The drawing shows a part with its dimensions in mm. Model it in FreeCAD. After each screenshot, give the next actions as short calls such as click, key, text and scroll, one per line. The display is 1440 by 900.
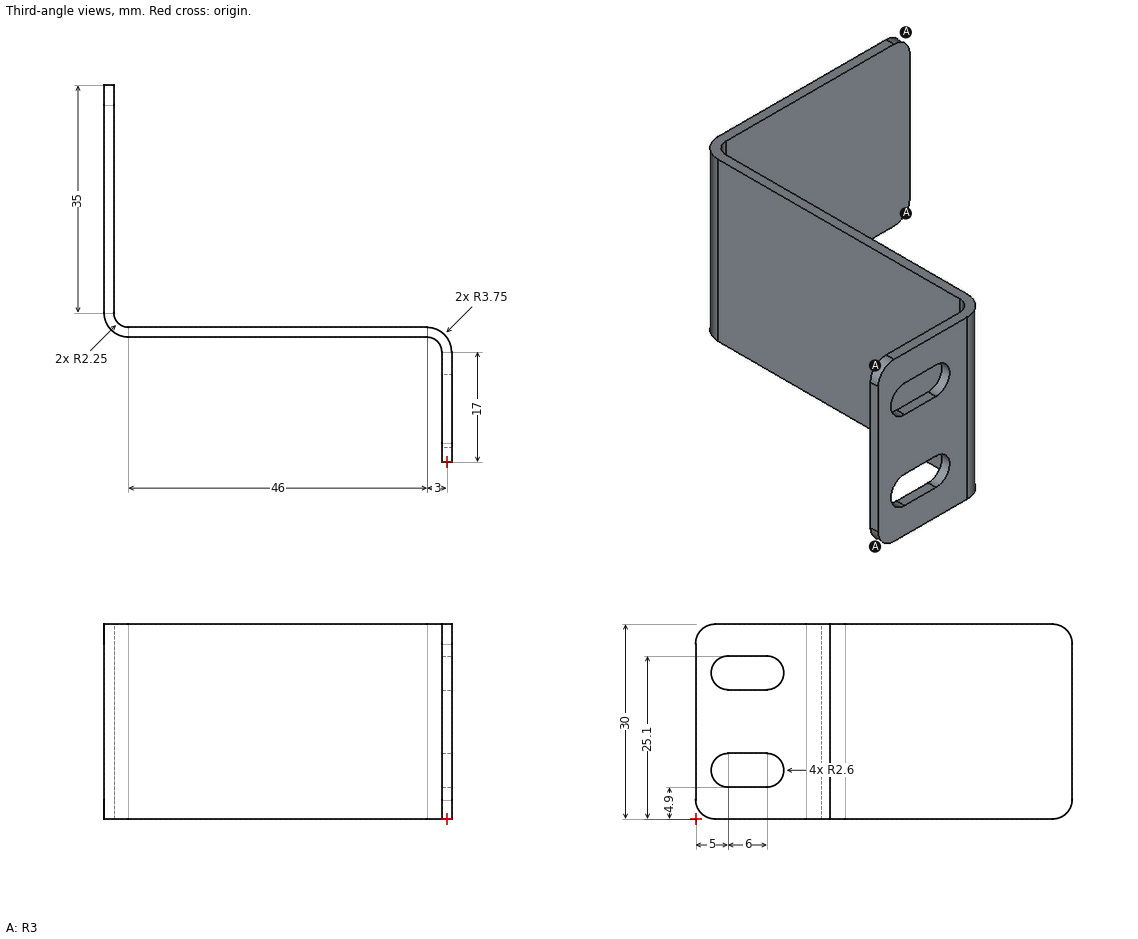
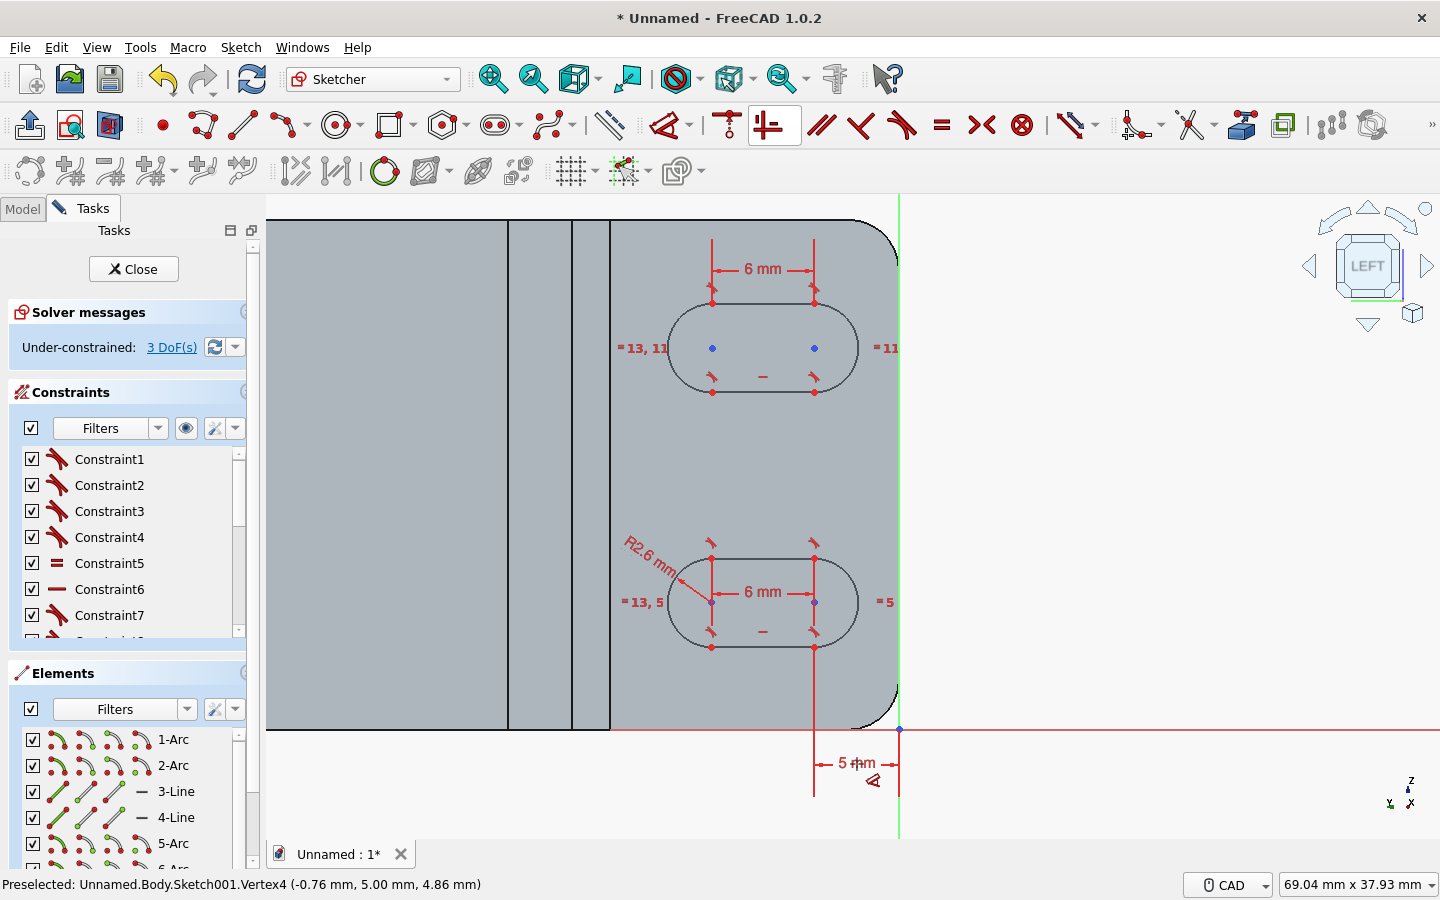
click(814, 392)
click(837, 358)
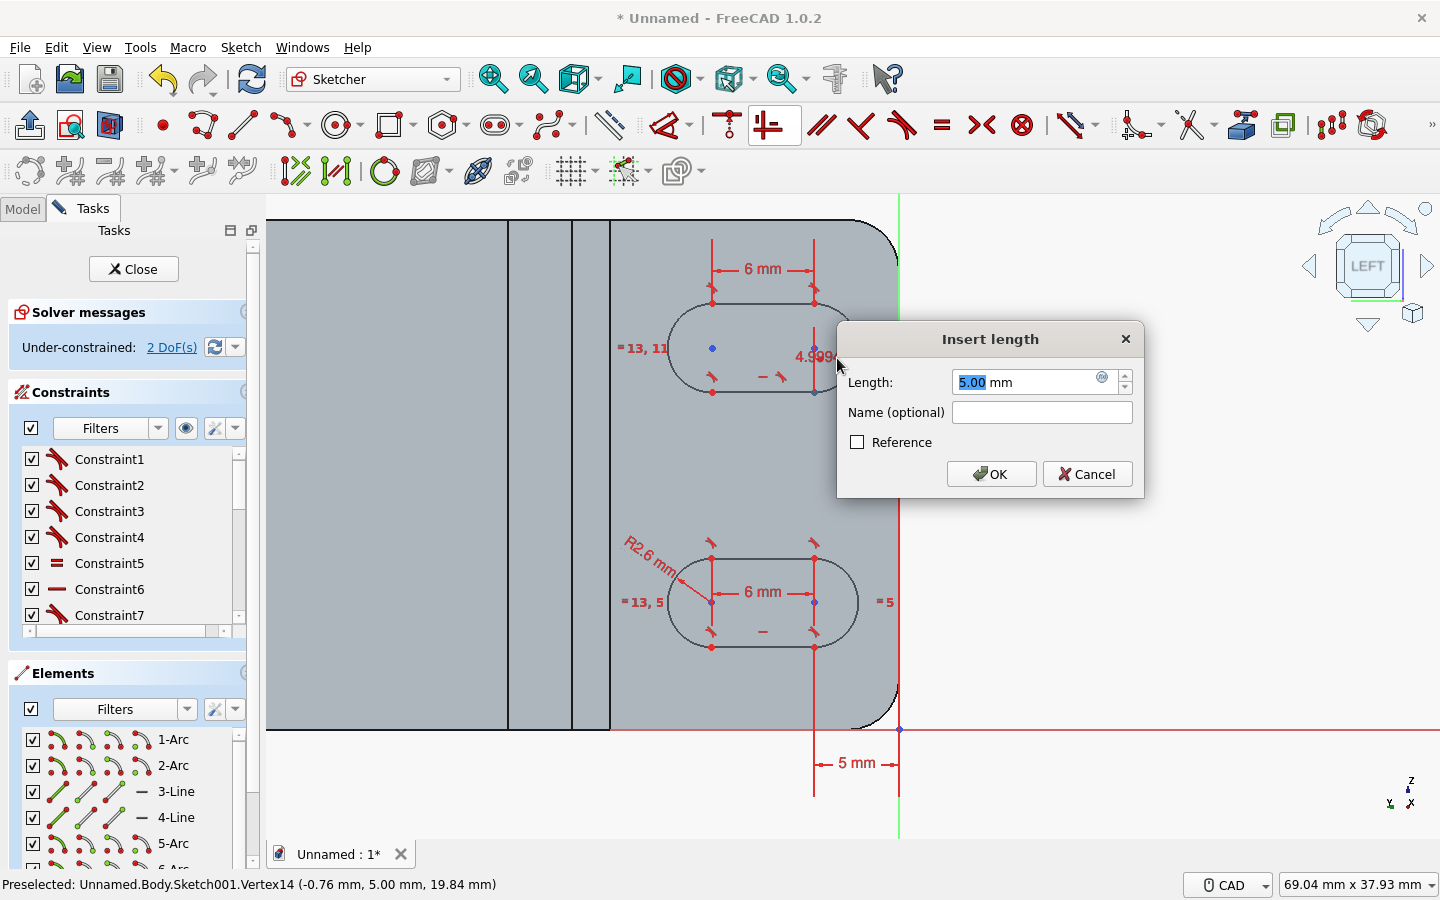
text(5)
key(Return)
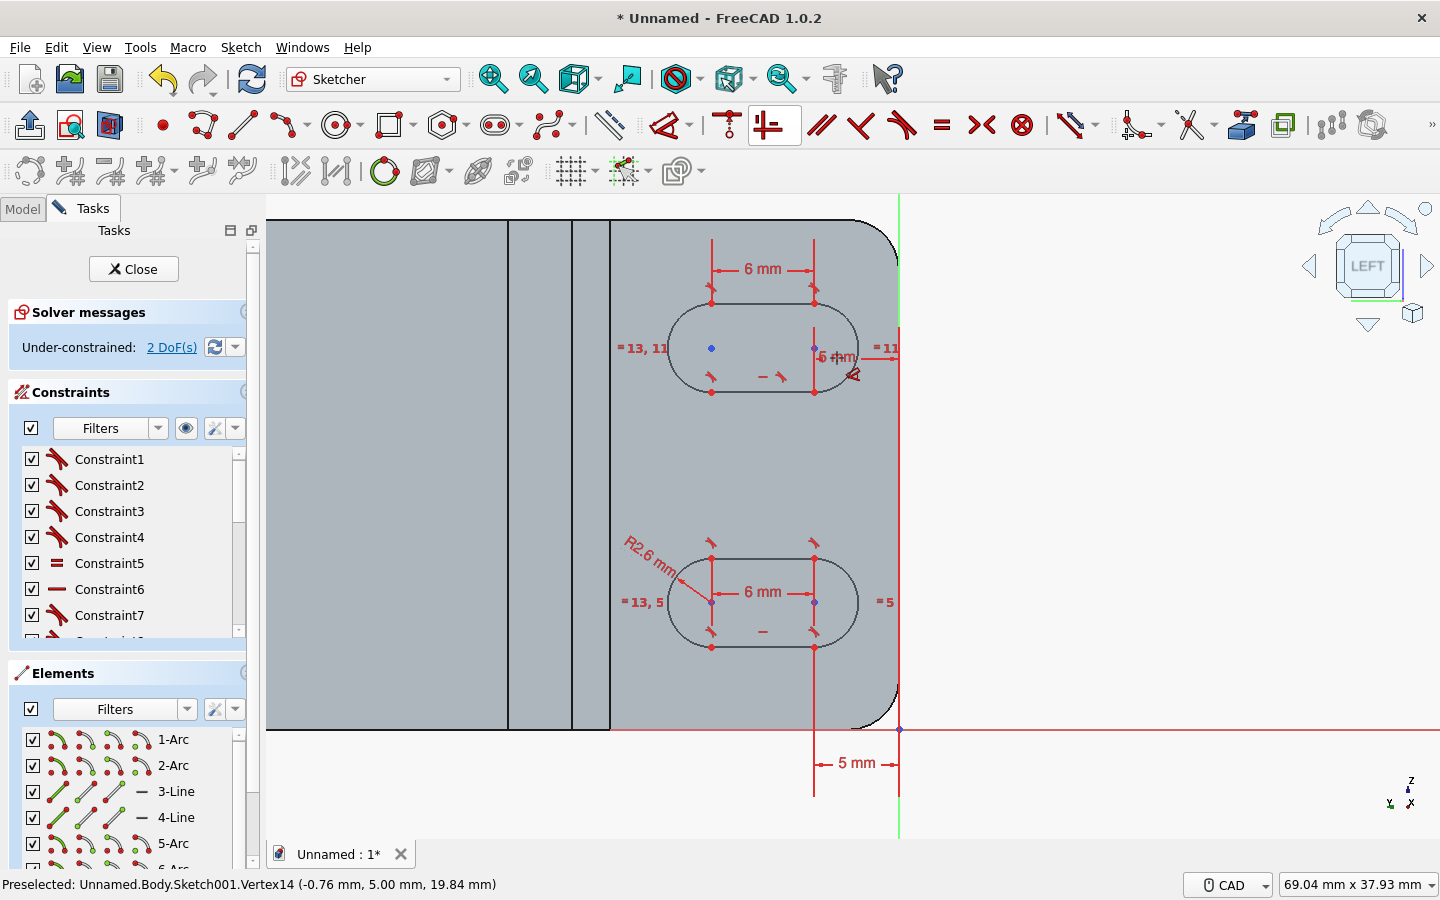
click(712, 647)
click(933, 689)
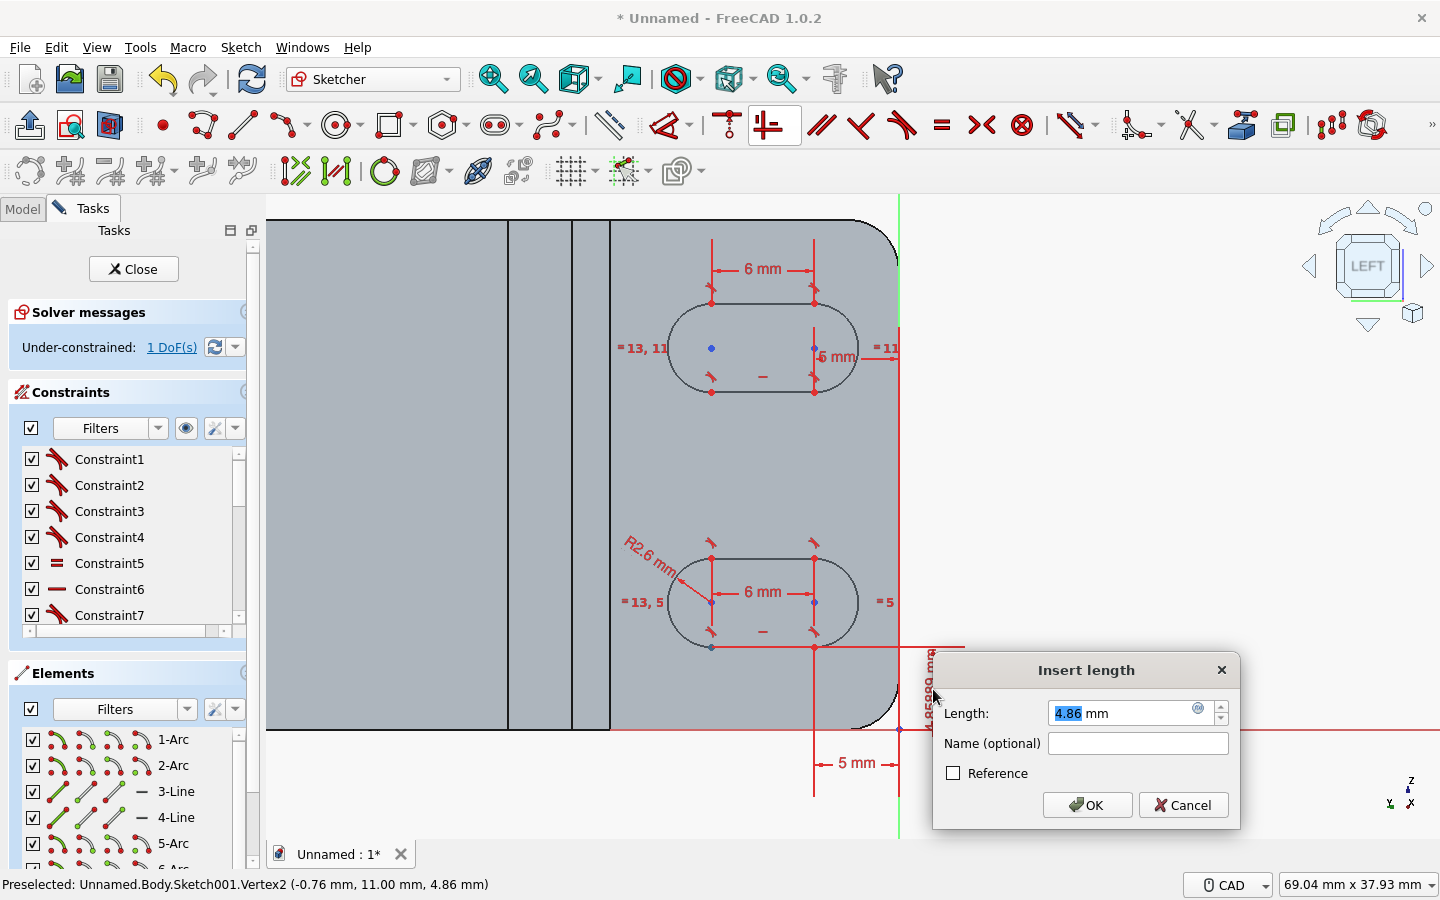
text(4.9)
key(Return)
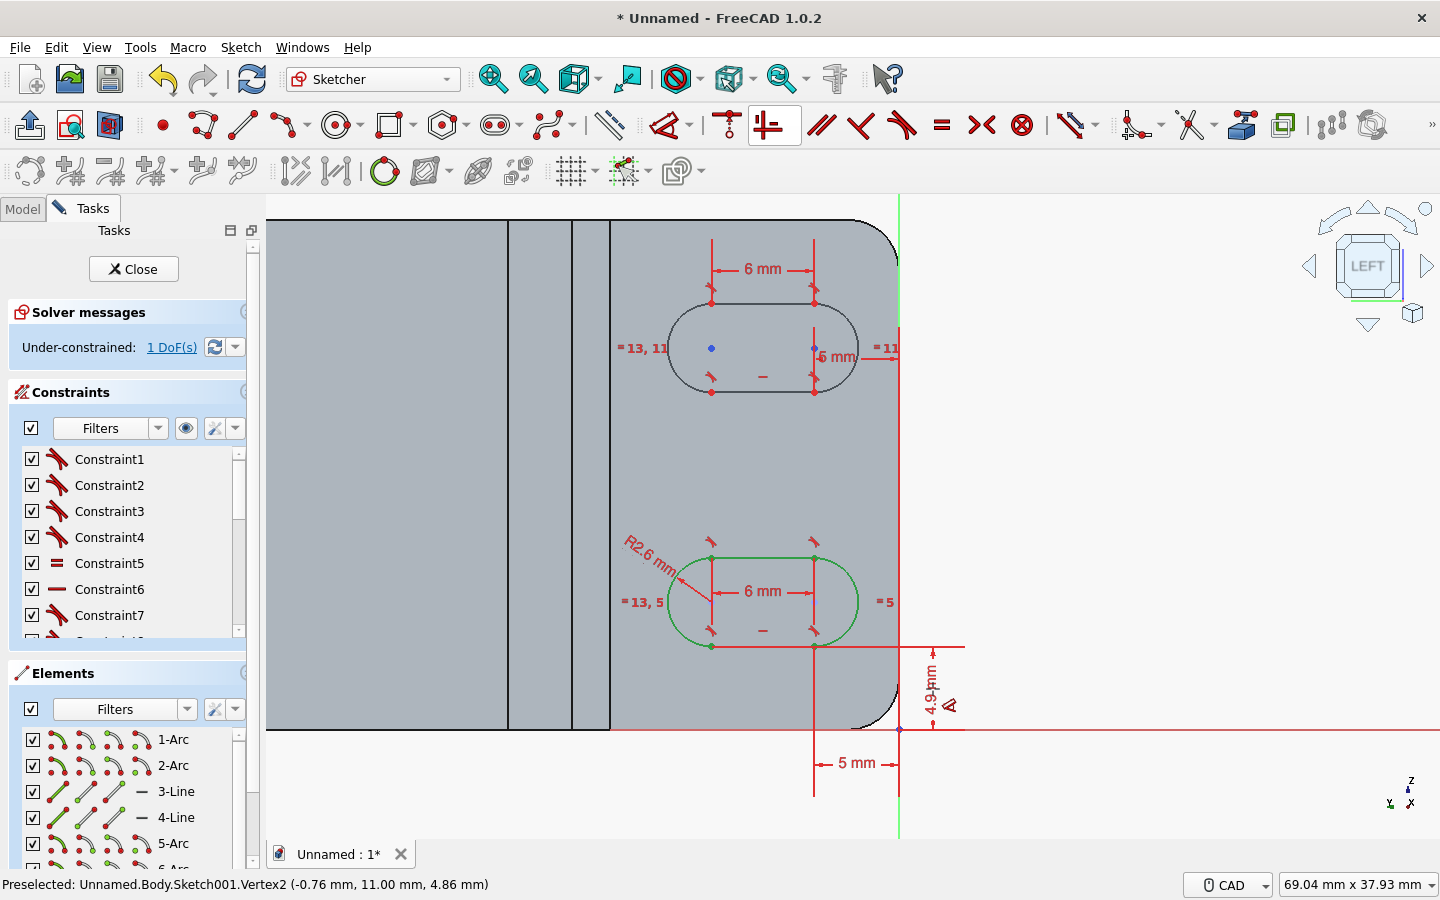
click(712, 304)
click(933, 517)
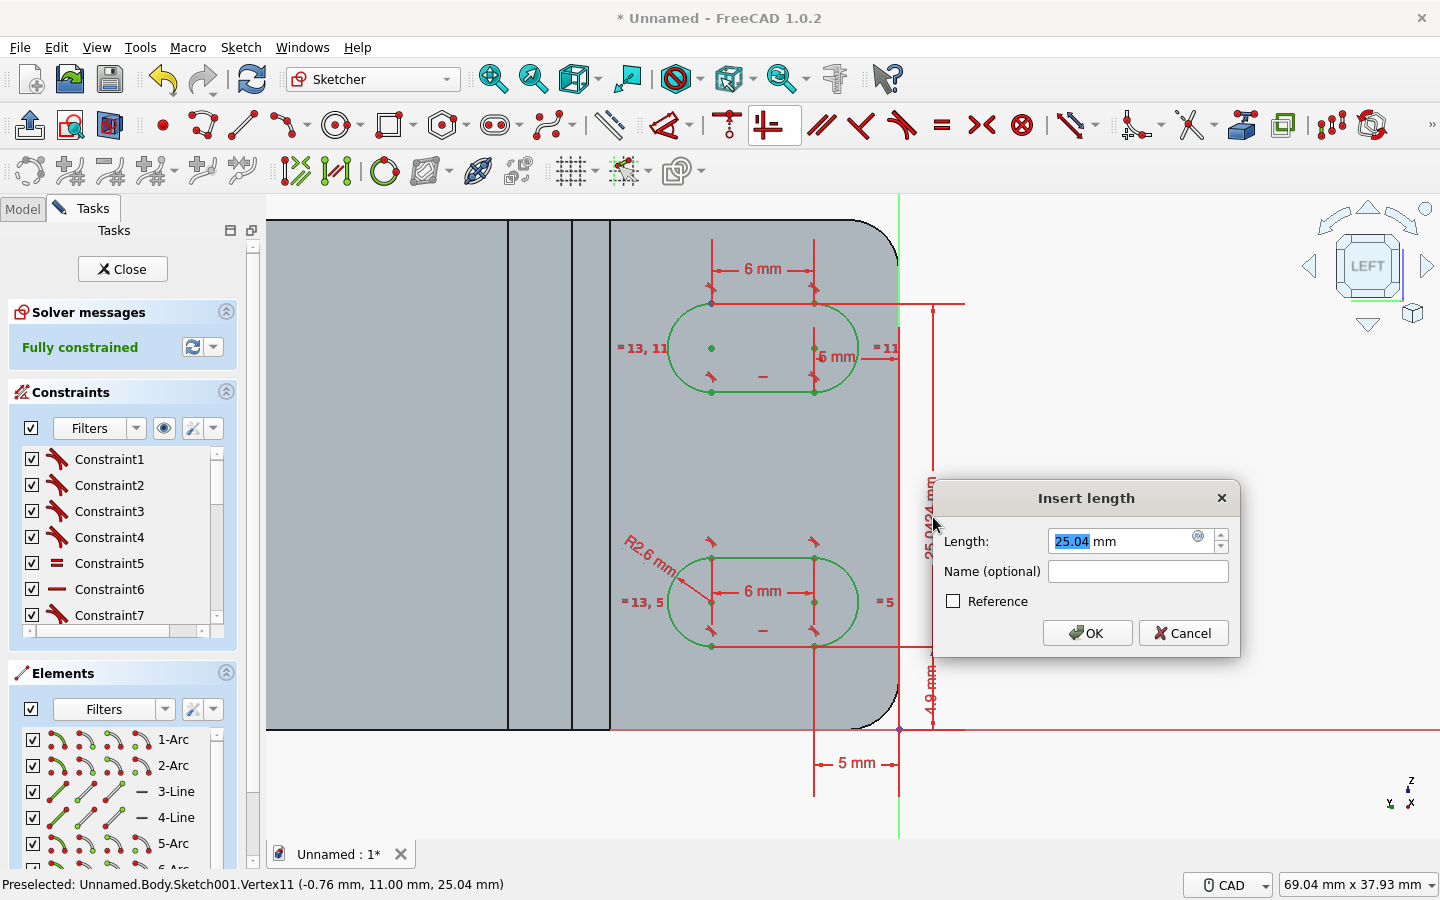
text(25.1)
key(Return)
key(Escape)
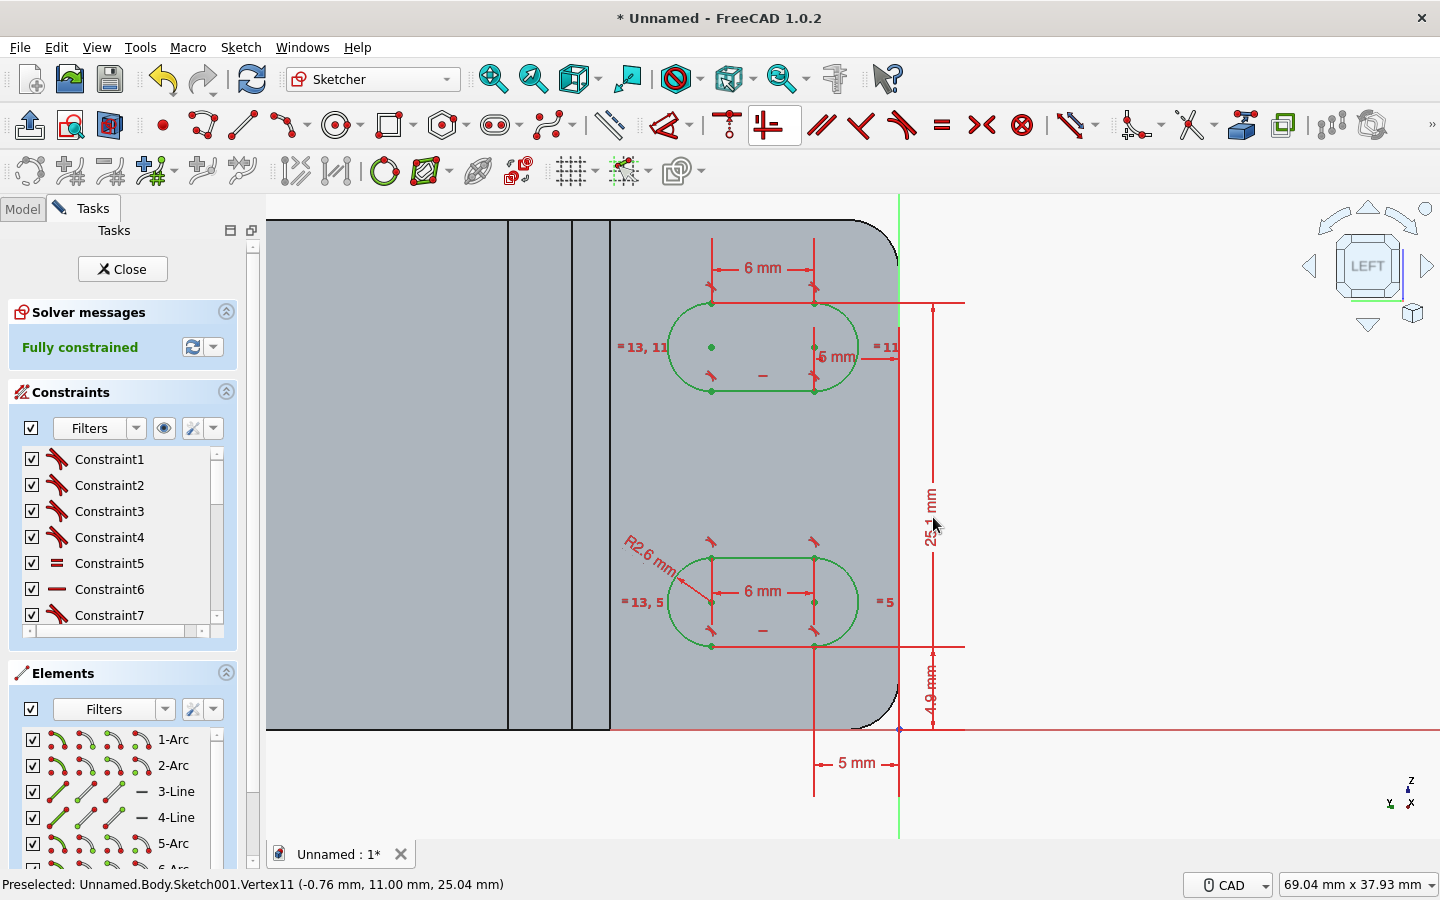
click(123, 269)